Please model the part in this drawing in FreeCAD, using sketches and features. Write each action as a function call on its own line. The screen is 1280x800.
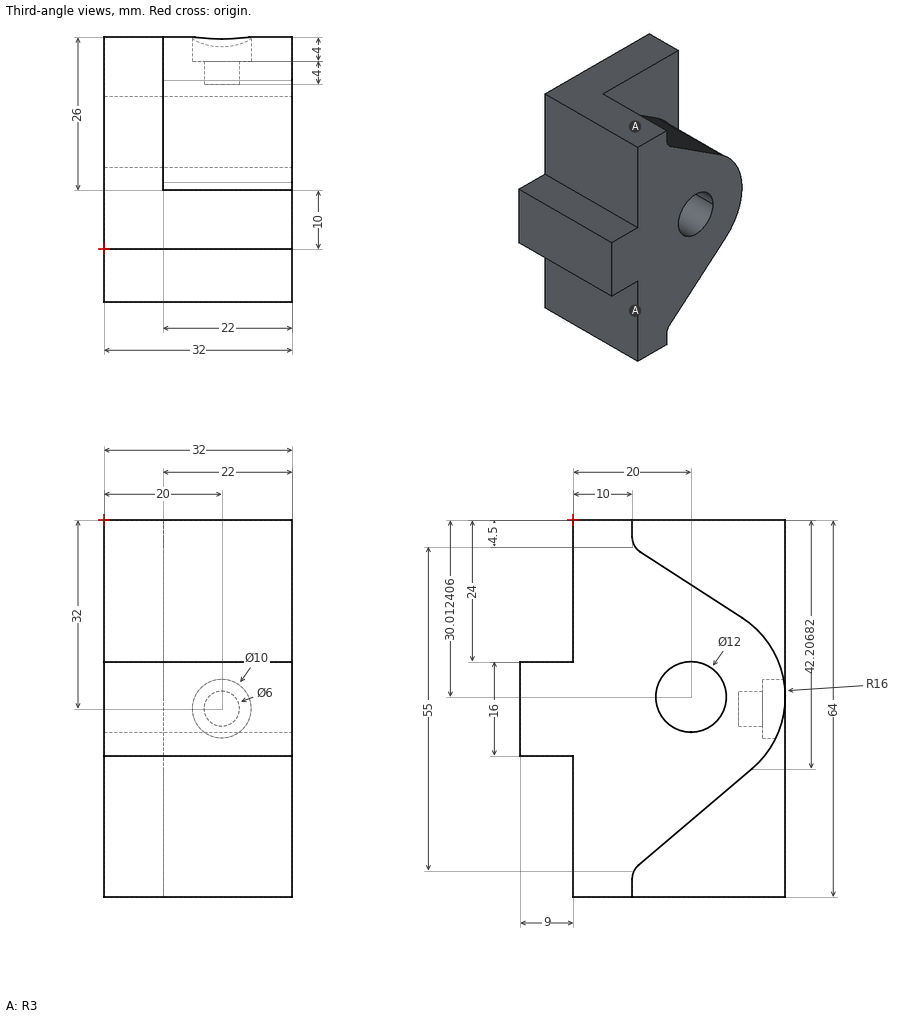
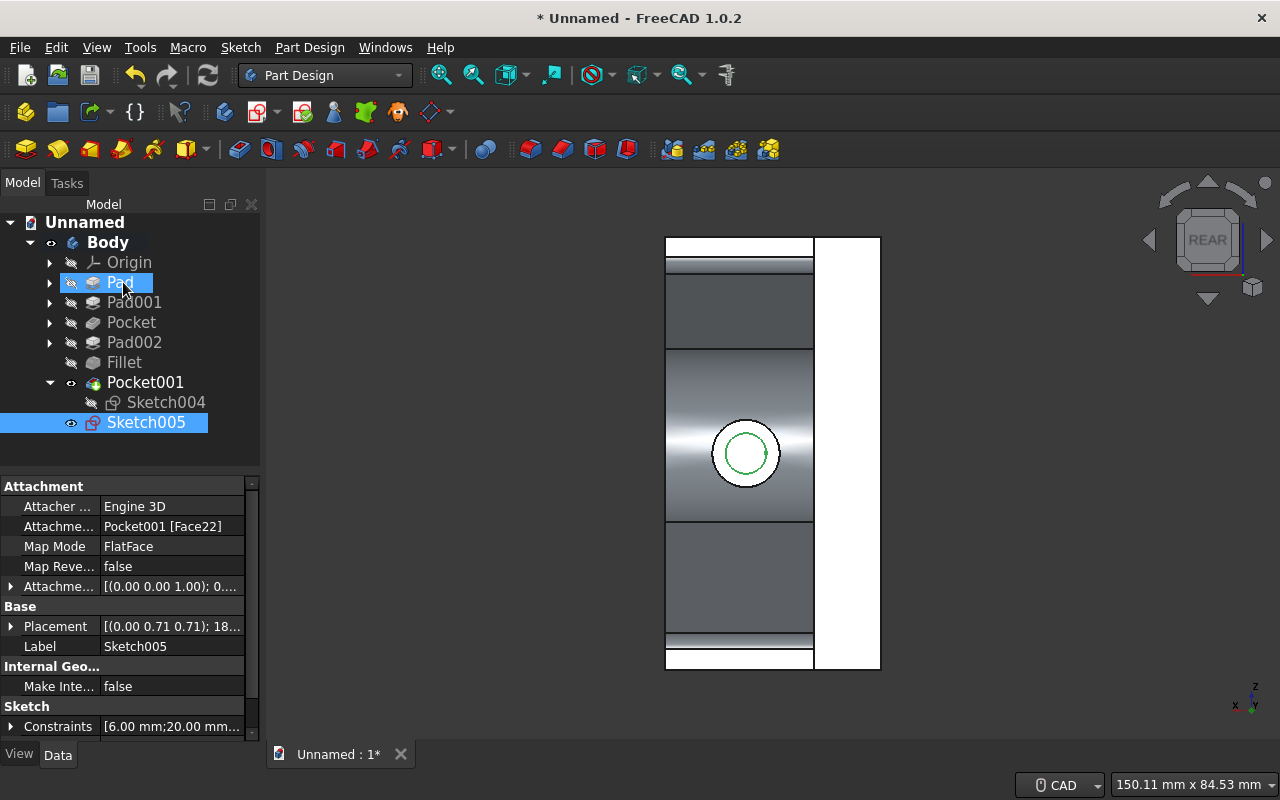
click(240, 150)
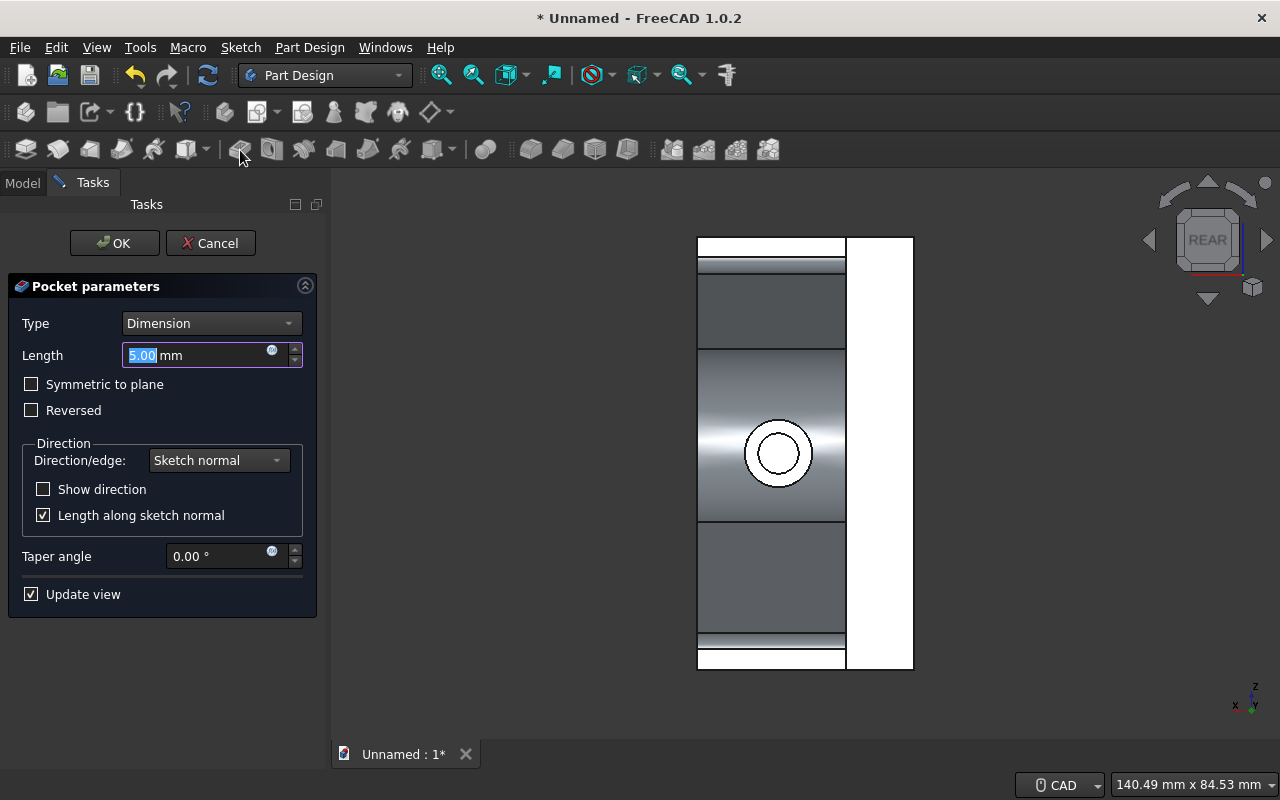
text(4)
key(Tab)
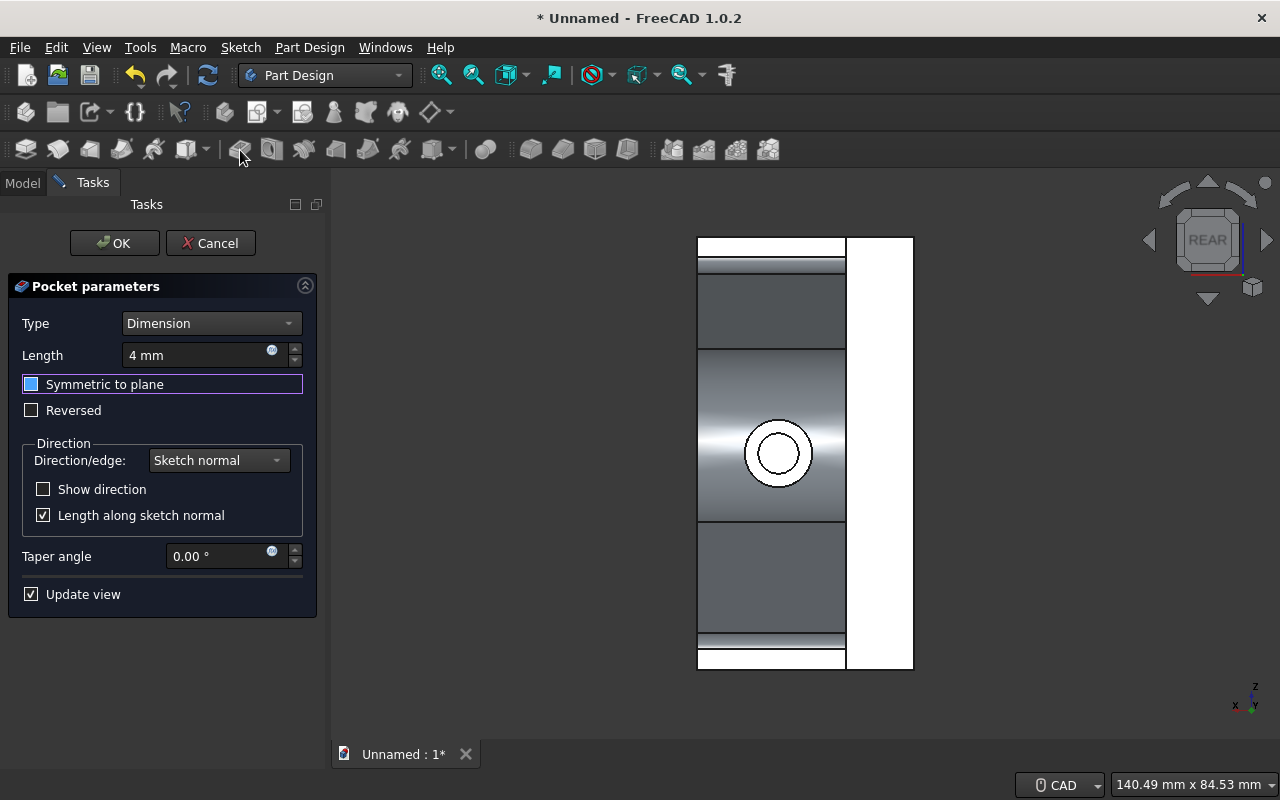
click(115, 243)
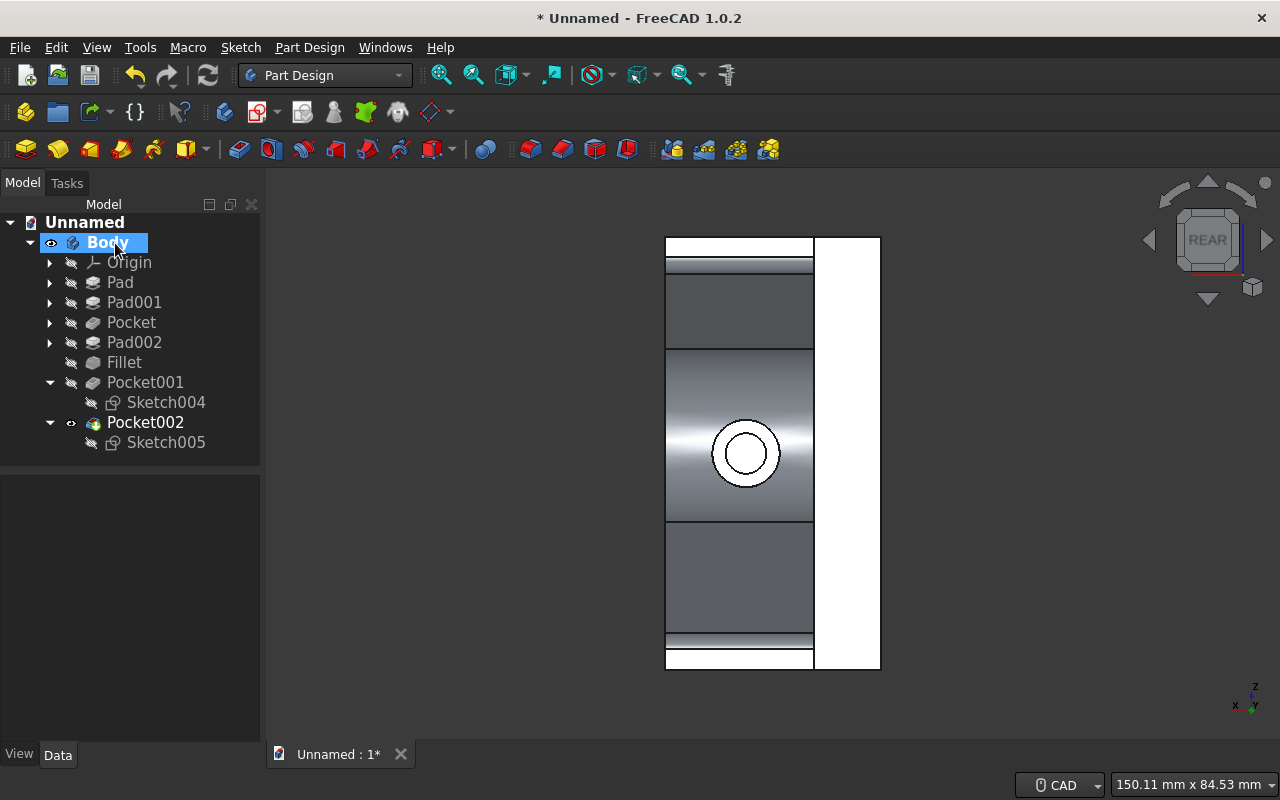
key(0)